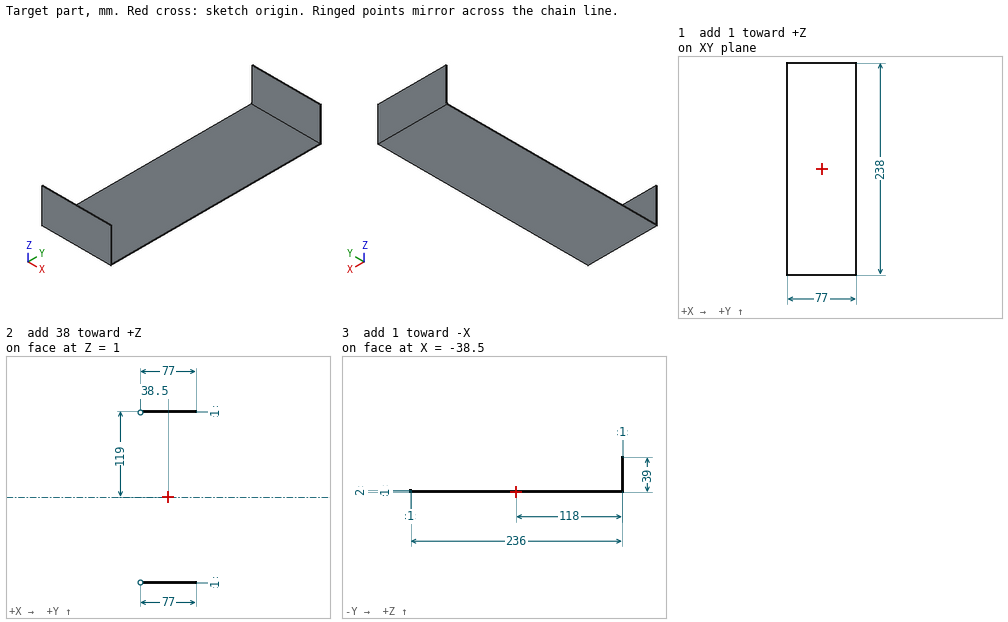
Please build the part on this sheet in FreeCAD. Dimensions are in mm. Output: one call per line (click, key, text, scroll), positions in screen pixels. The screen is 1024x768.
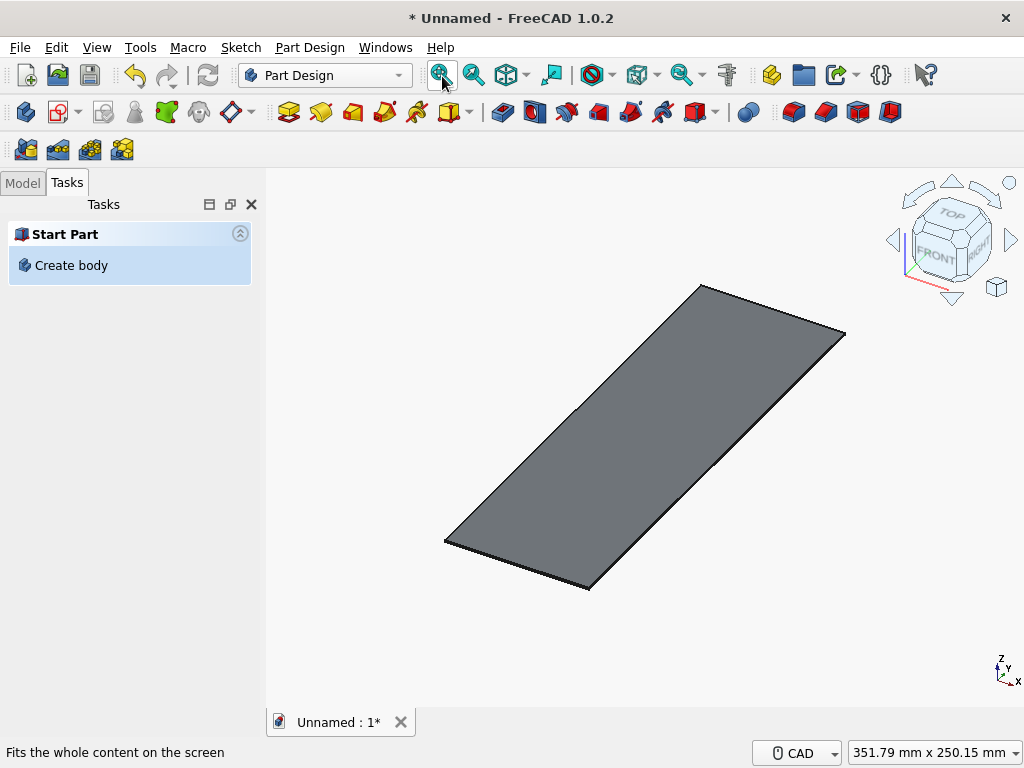
click(718, 363)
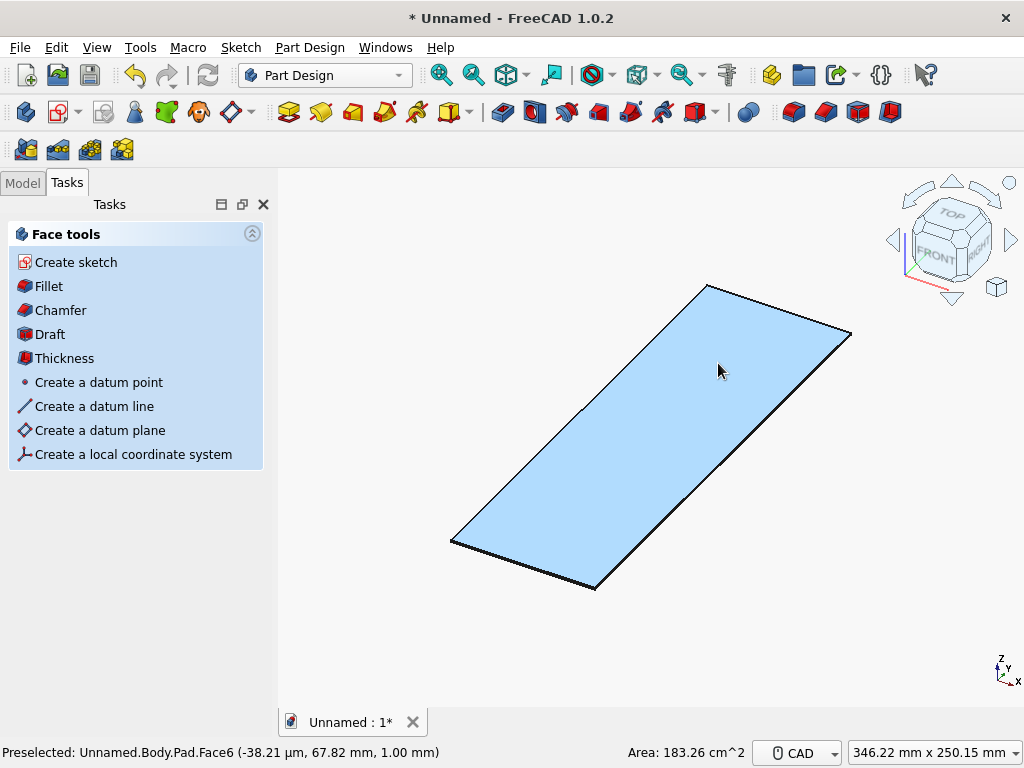
click(58, 112)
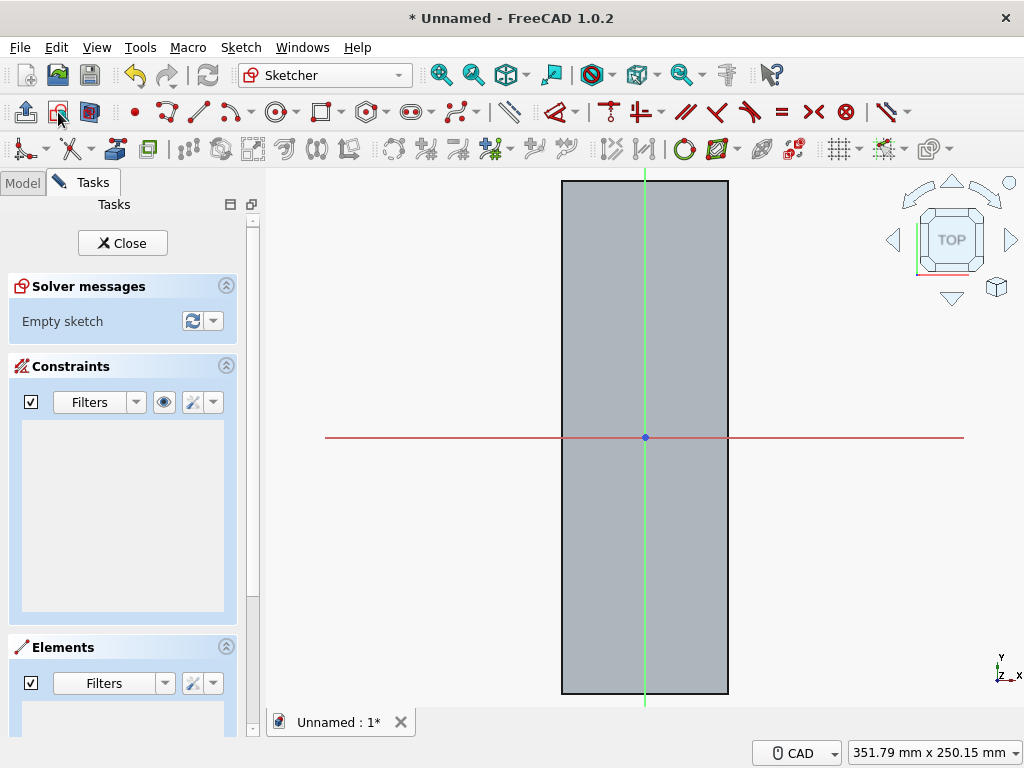
scroll(437, 438, down, 2)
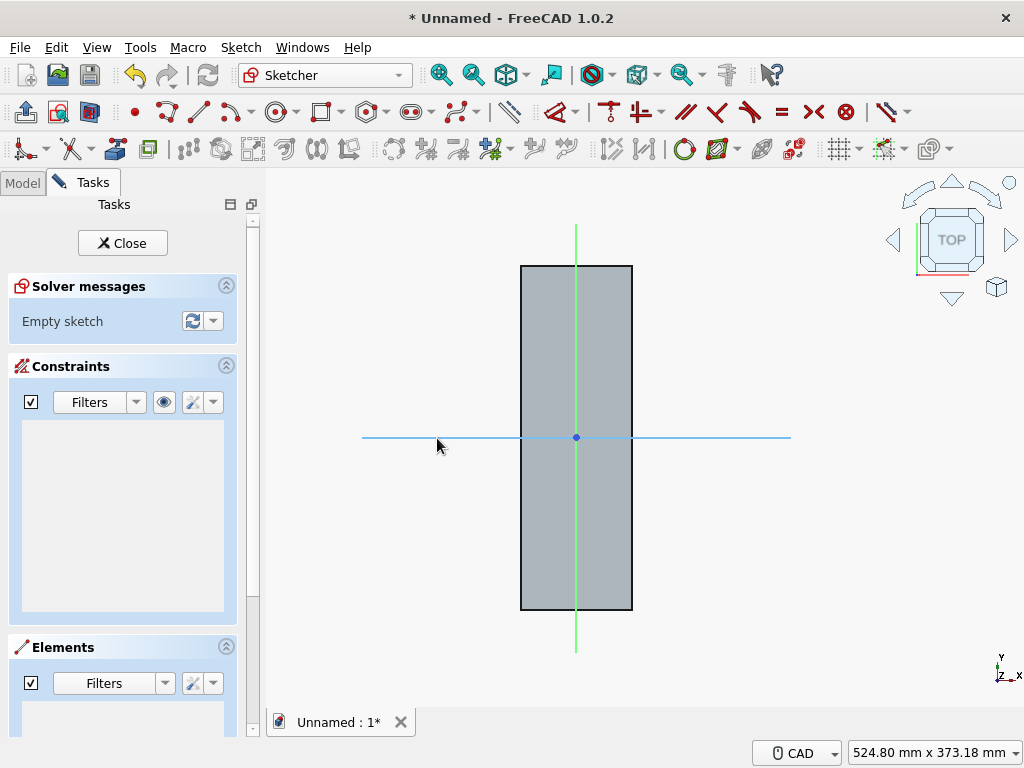
click(322, 112)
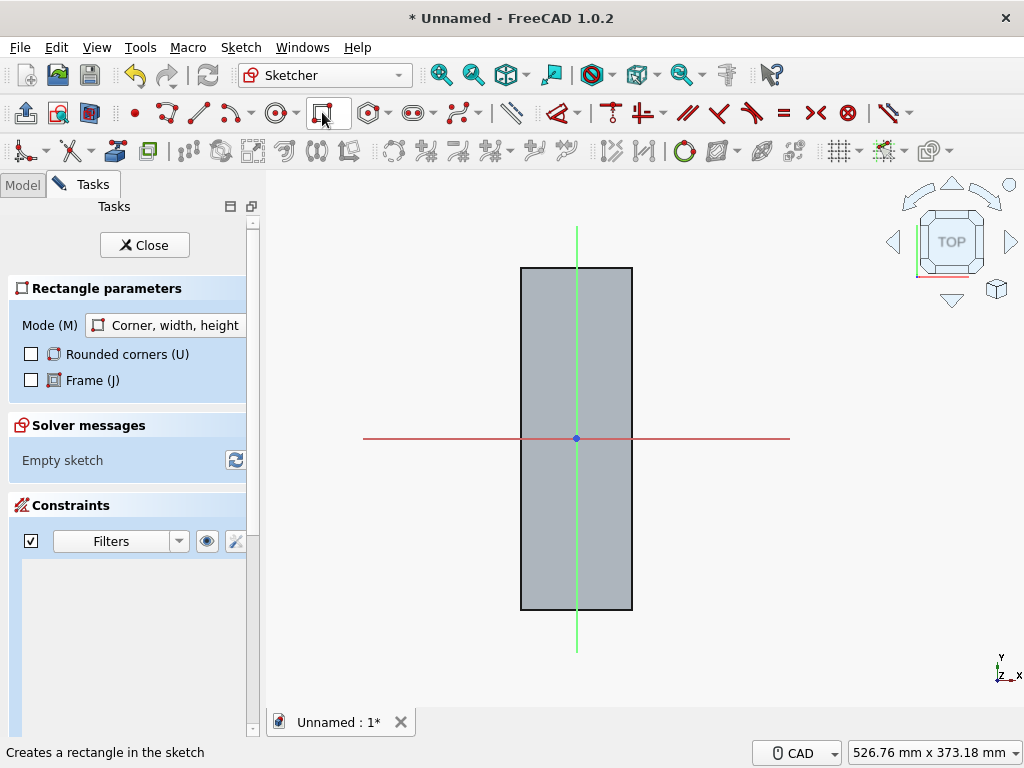
scroll(521, 268, up, 13)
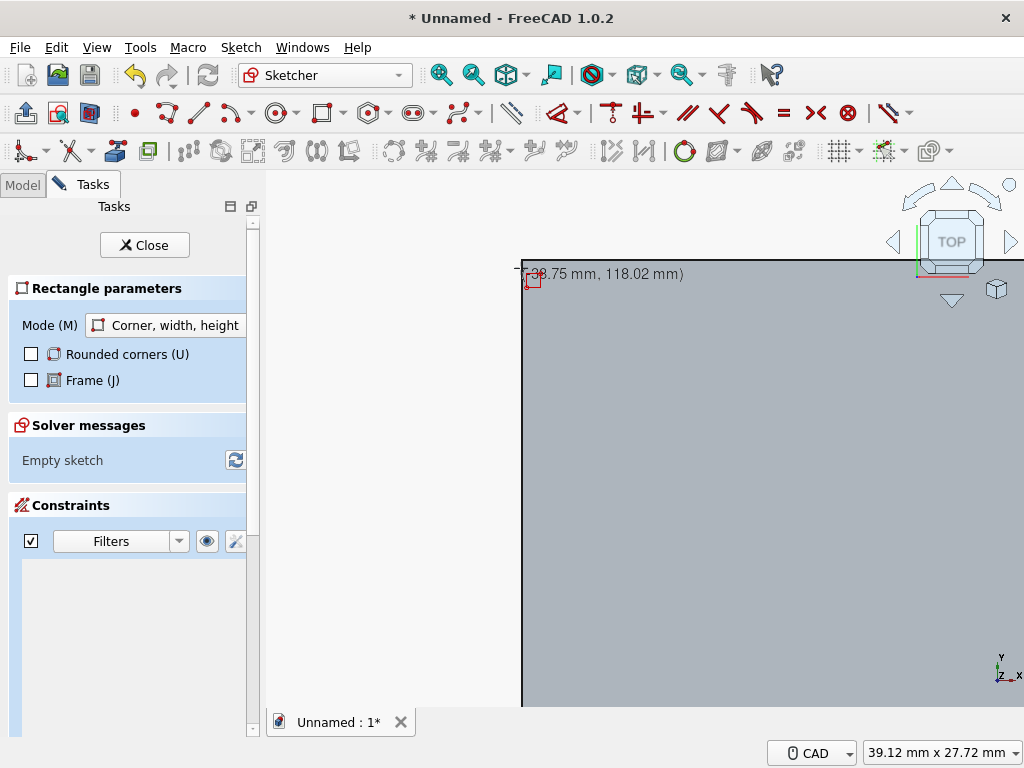
scroll(521, 268, down, 13)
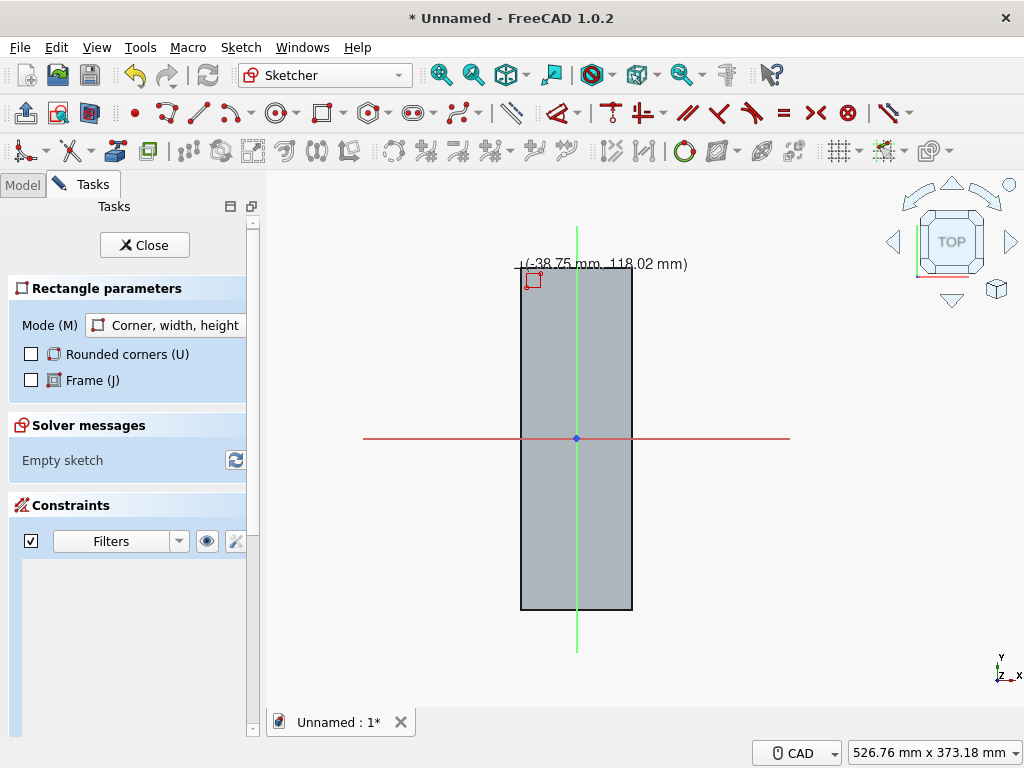
click(521, 268)
move(632, 269)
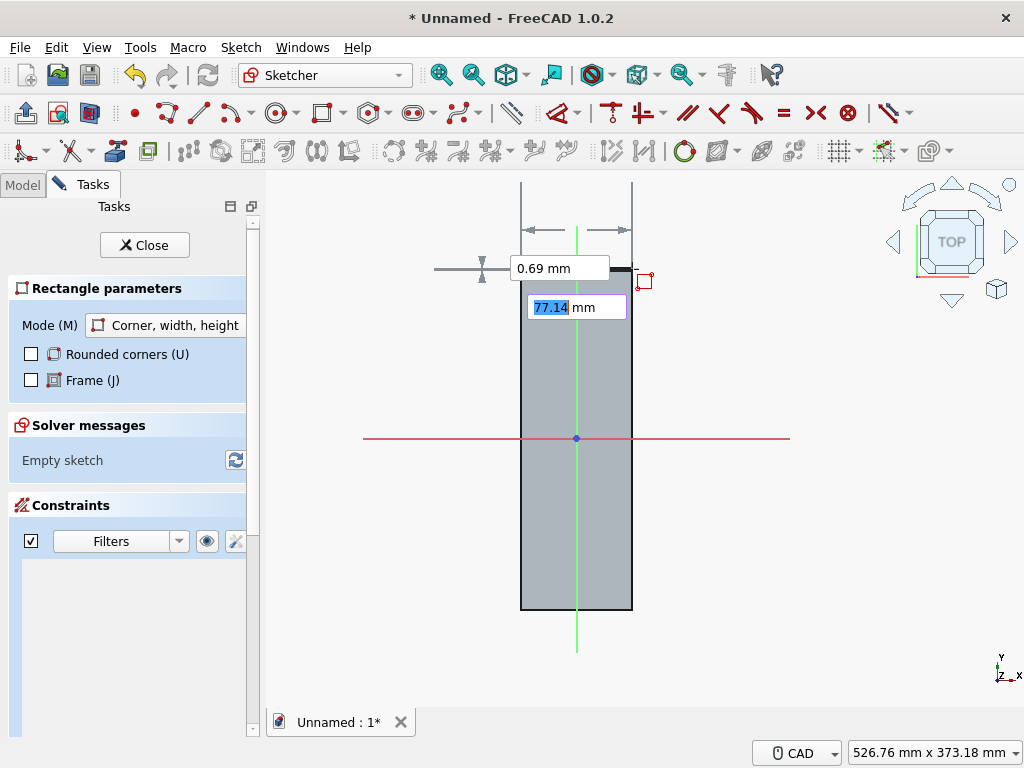
text(77)
key(Tab)
text(1)
key(Return)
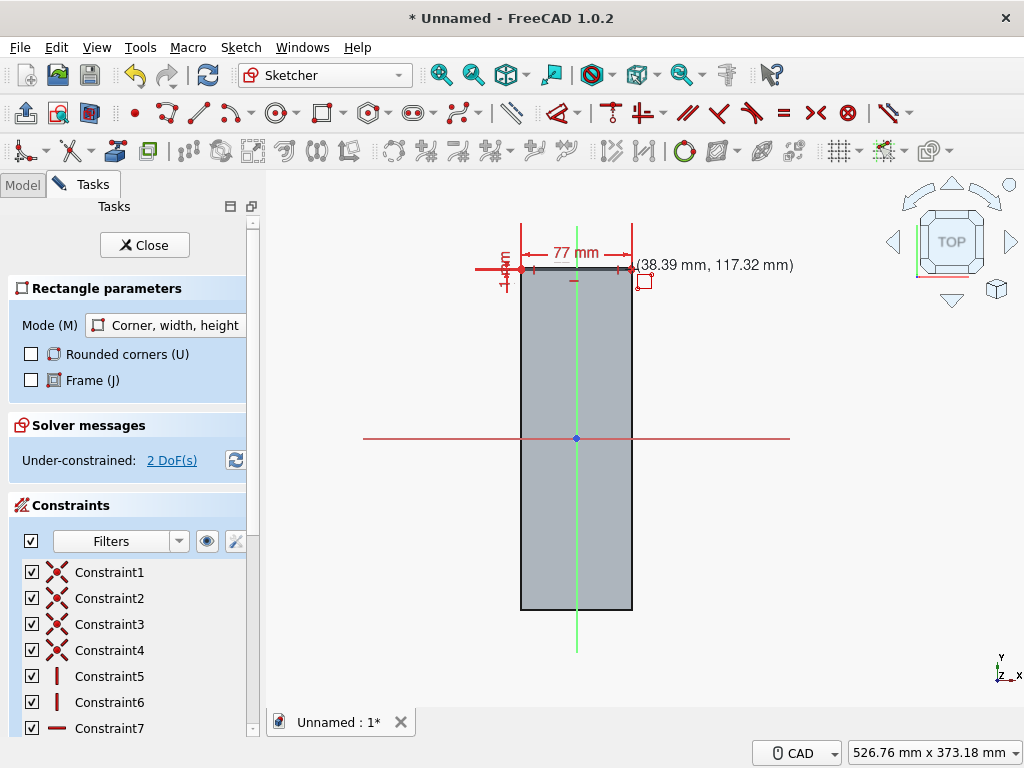
scroll(521, 609, up, 13)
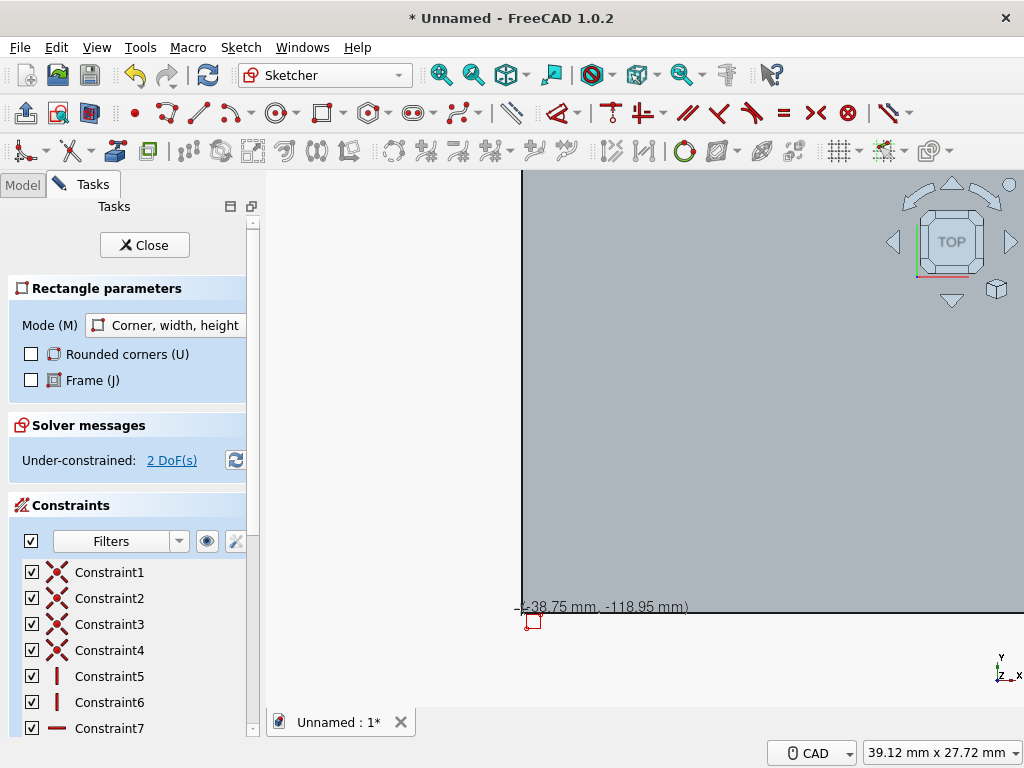
scroll(521, 609, down, 13)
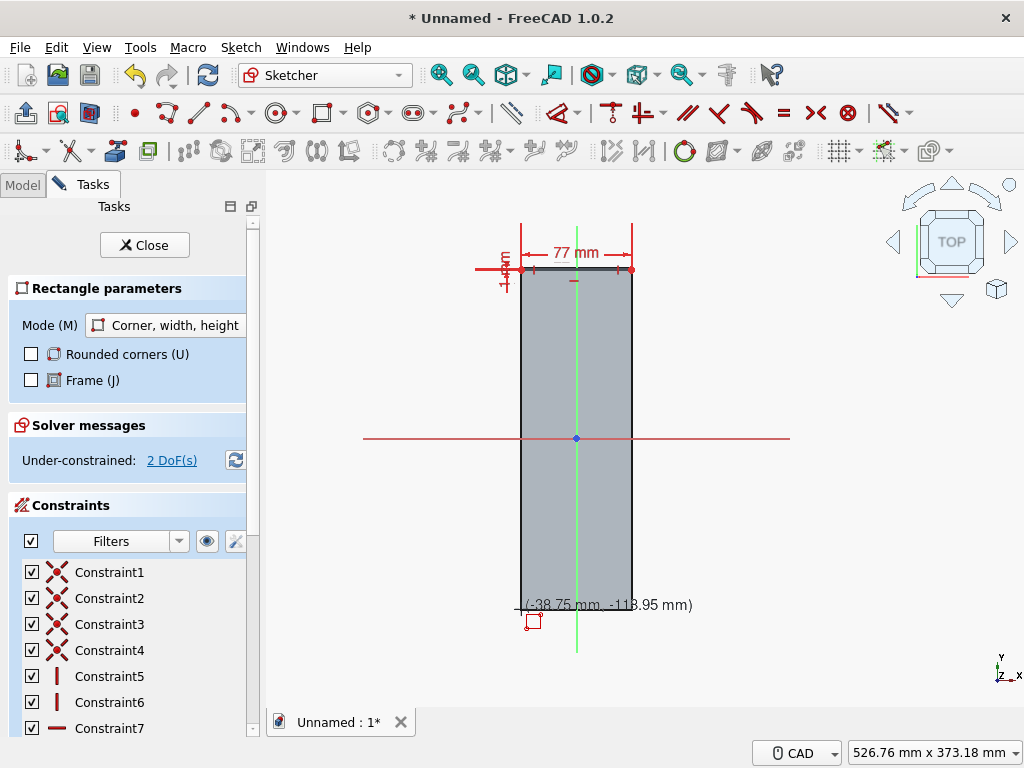
click(521, 609)
move(632, 610)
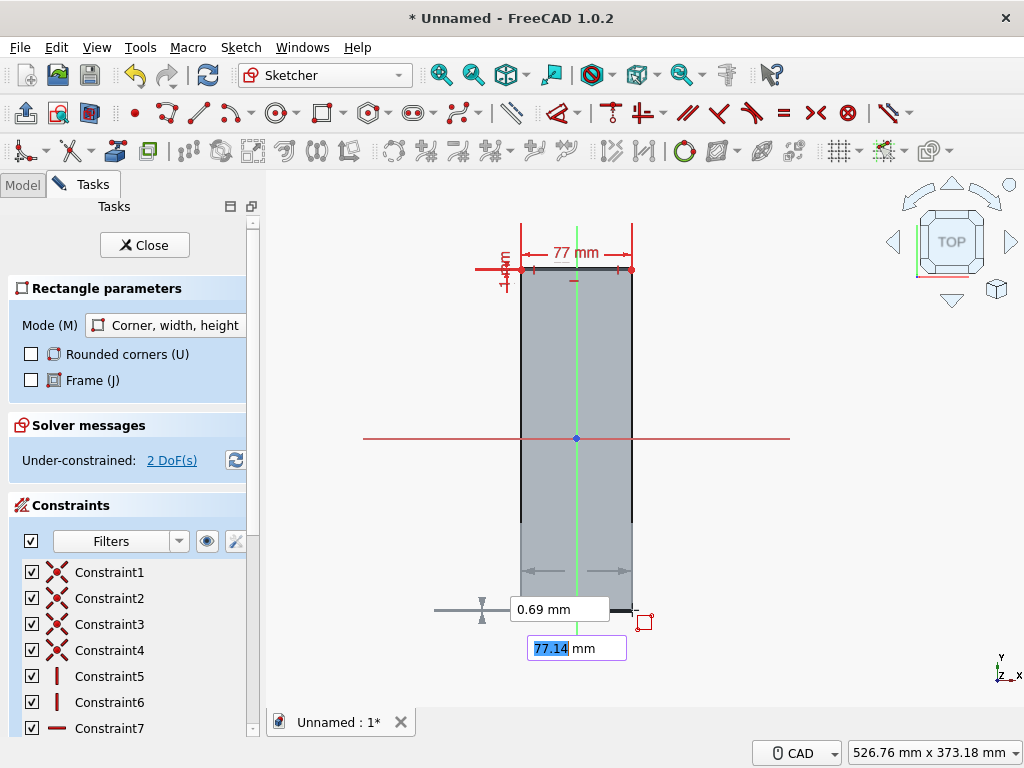
text(77)
key(Tab)
text(1)
key(Return)
key(Escape)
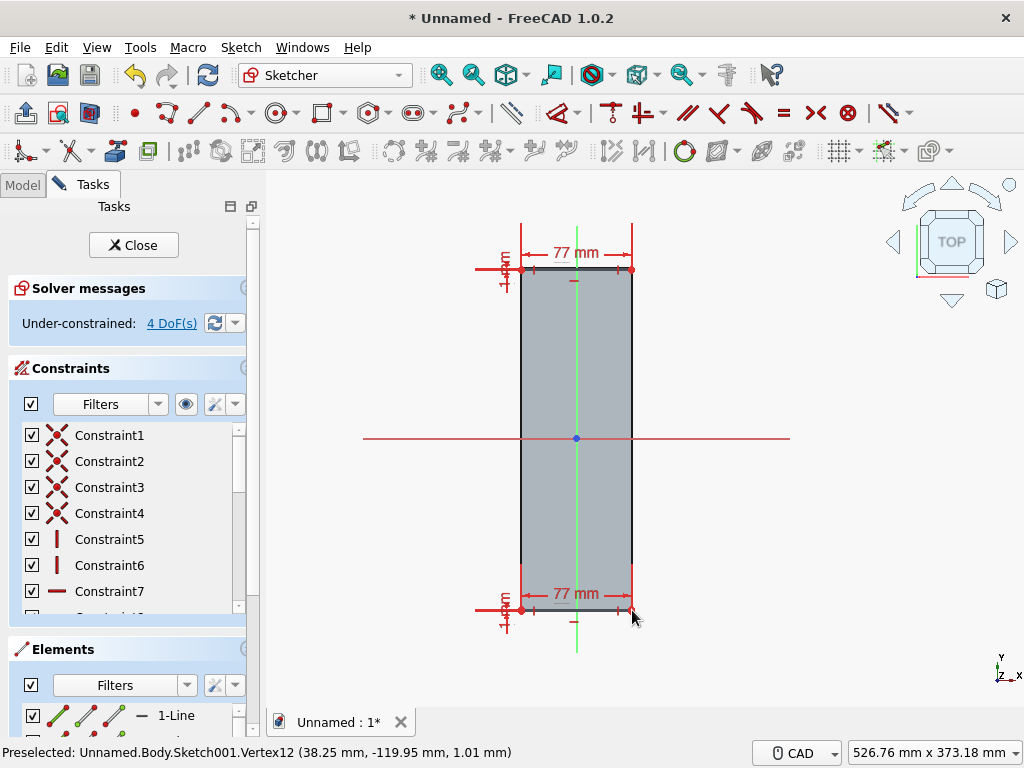
scroll(521, 270, up, 11)